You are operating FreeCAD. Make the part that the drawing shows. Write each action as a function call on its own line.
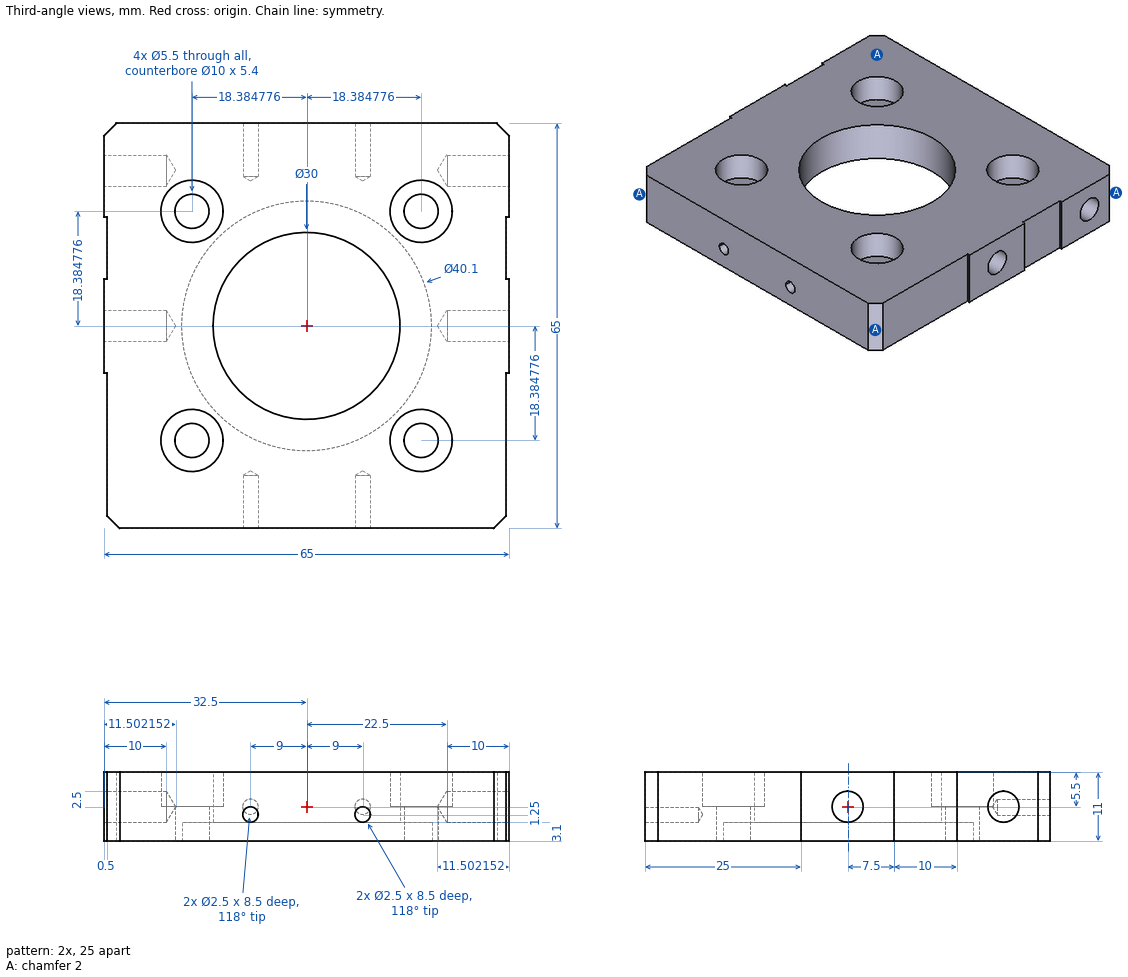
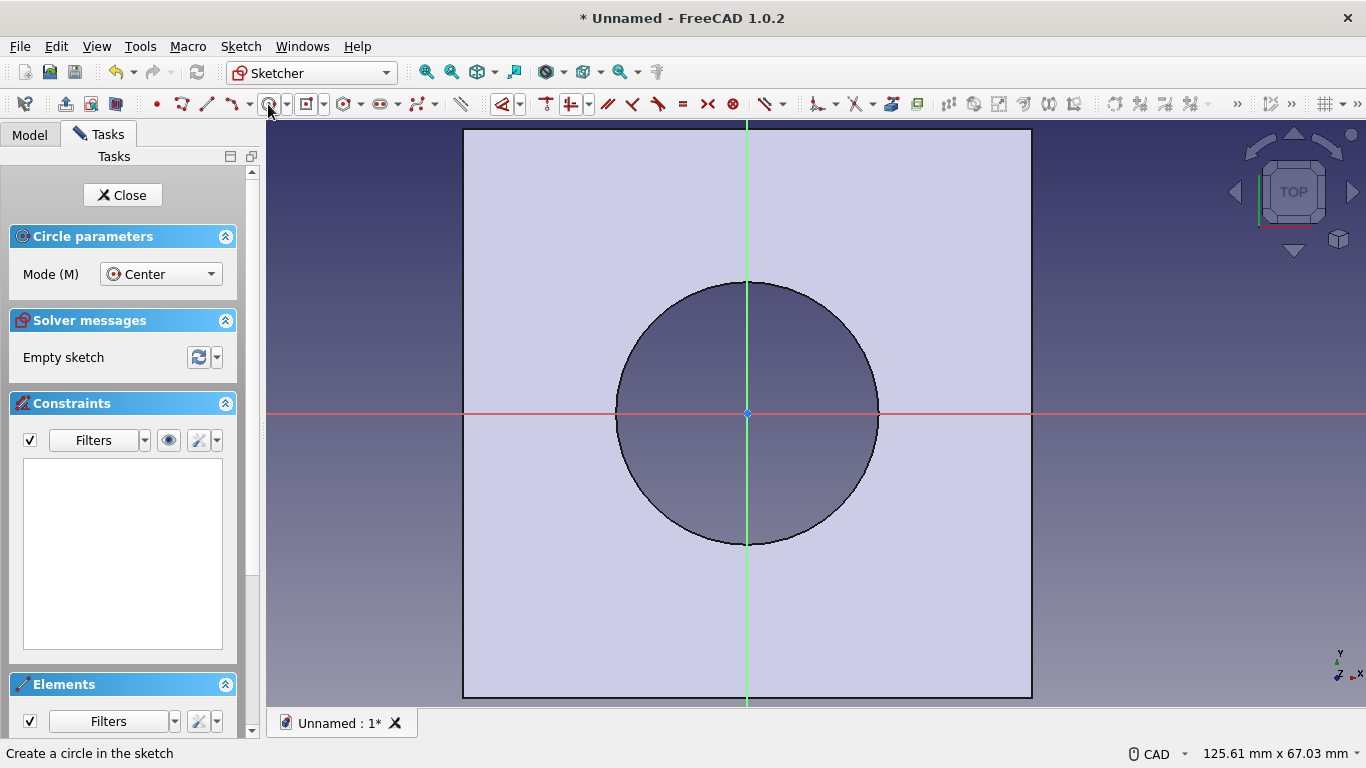
click(586, 253)
click(603, 235)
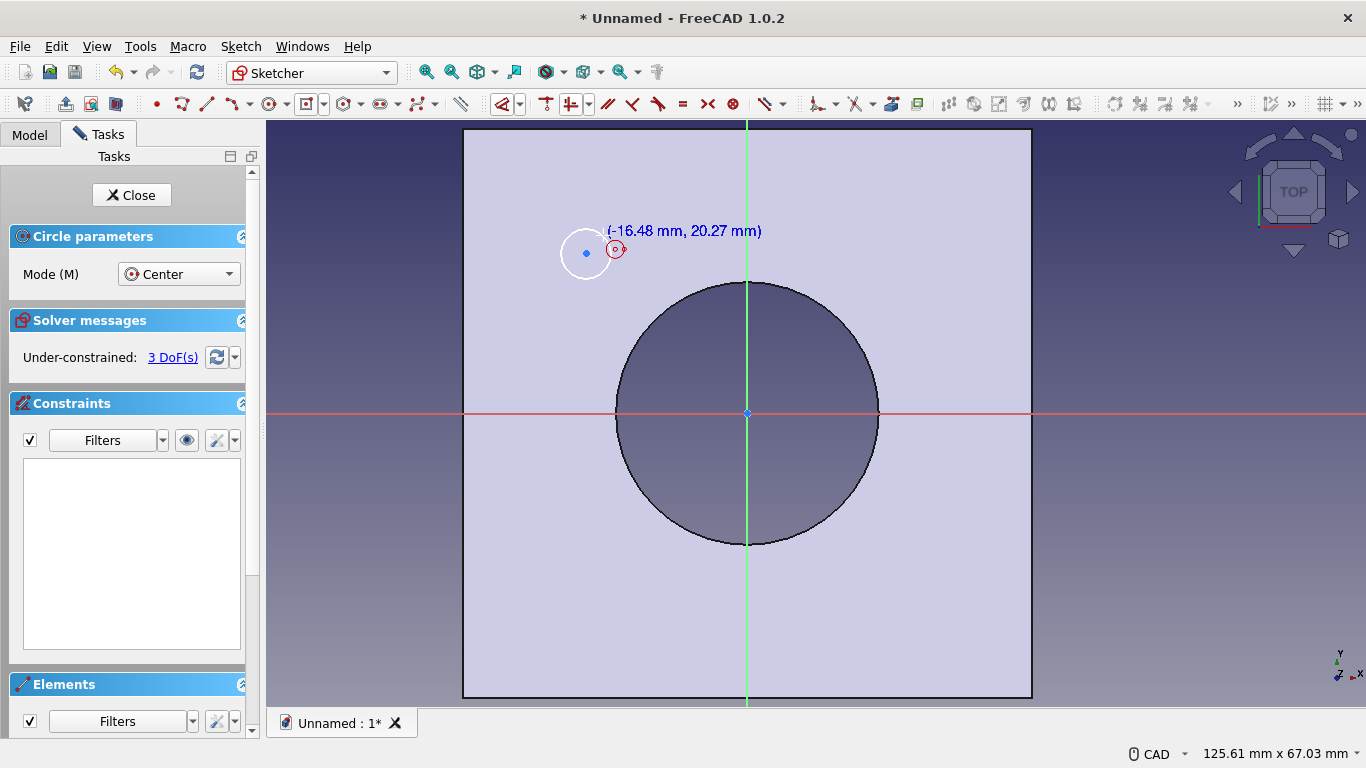
click(908, 253)
click(925, 235)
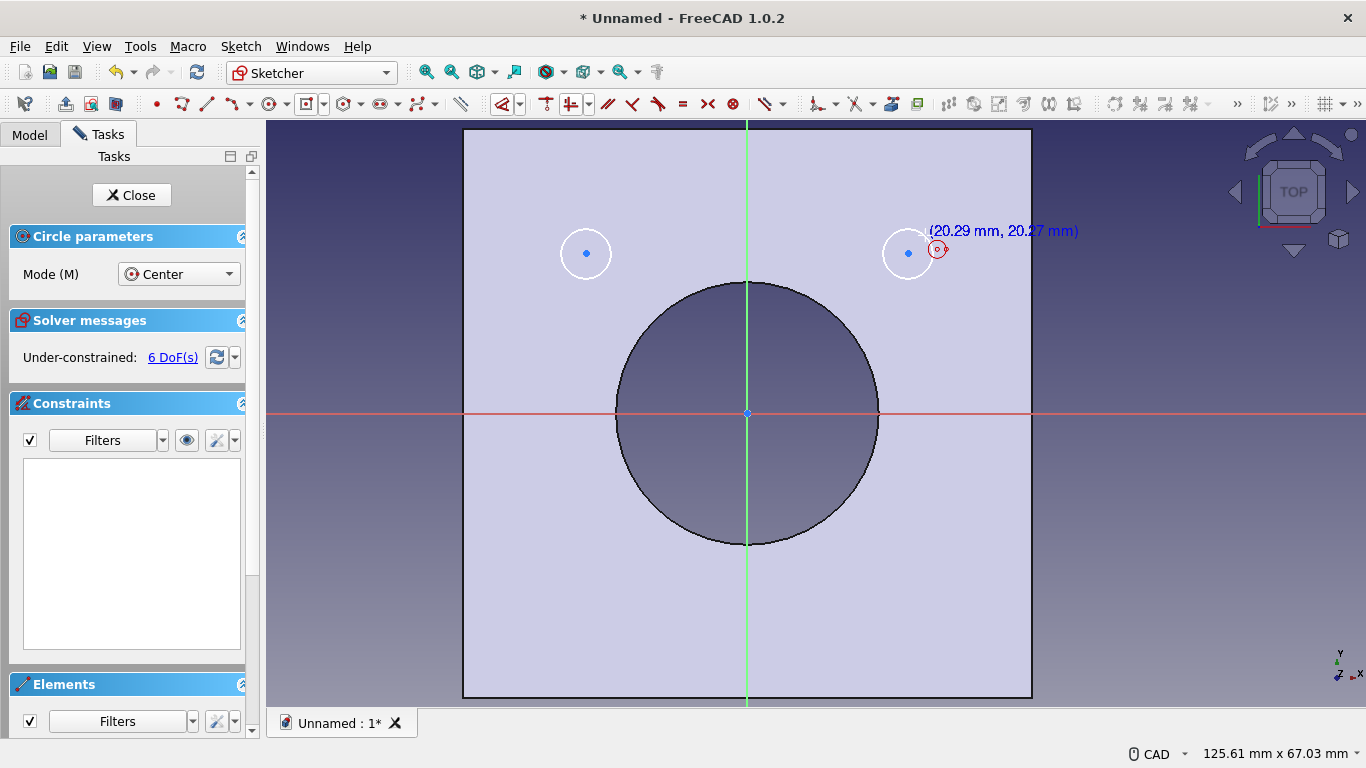
click(908, 574)
click(925, 557)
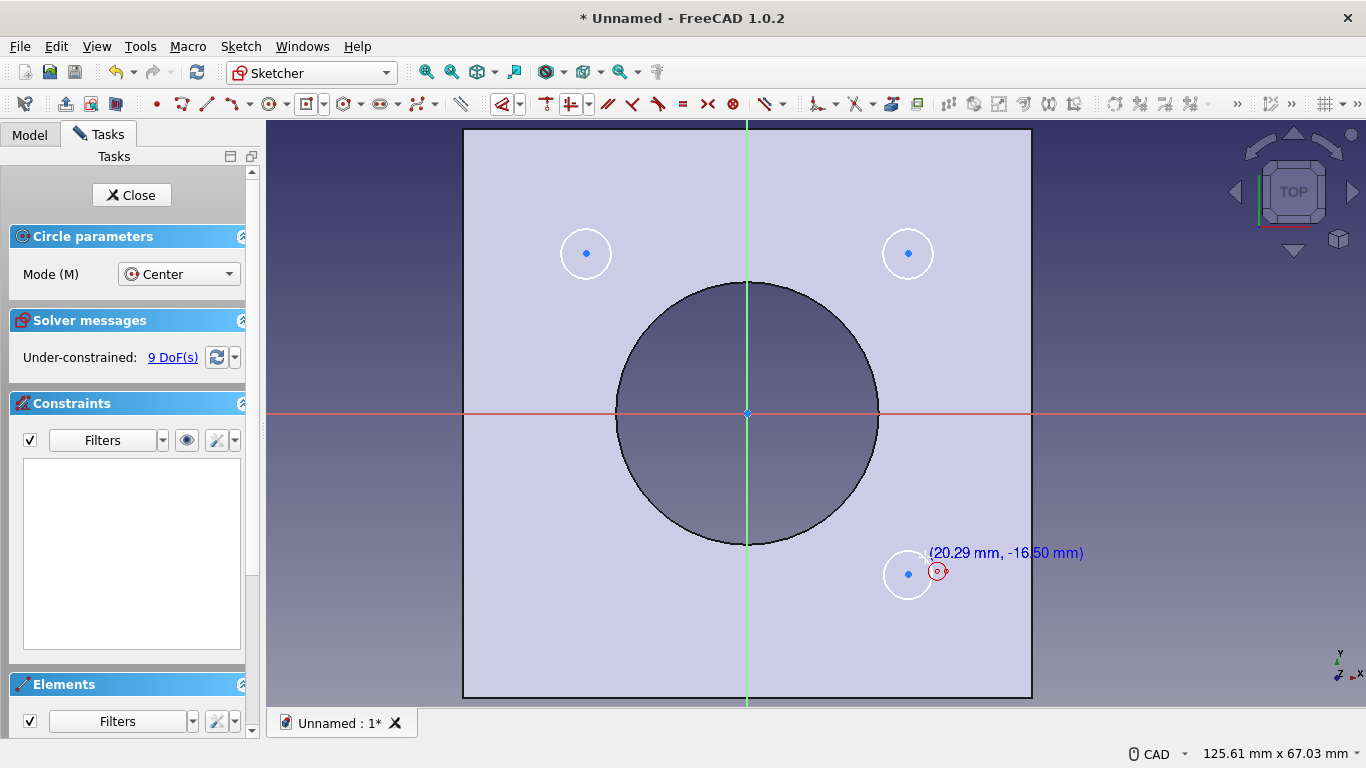
click(586, 574)
click(603, 557)
key(Escape)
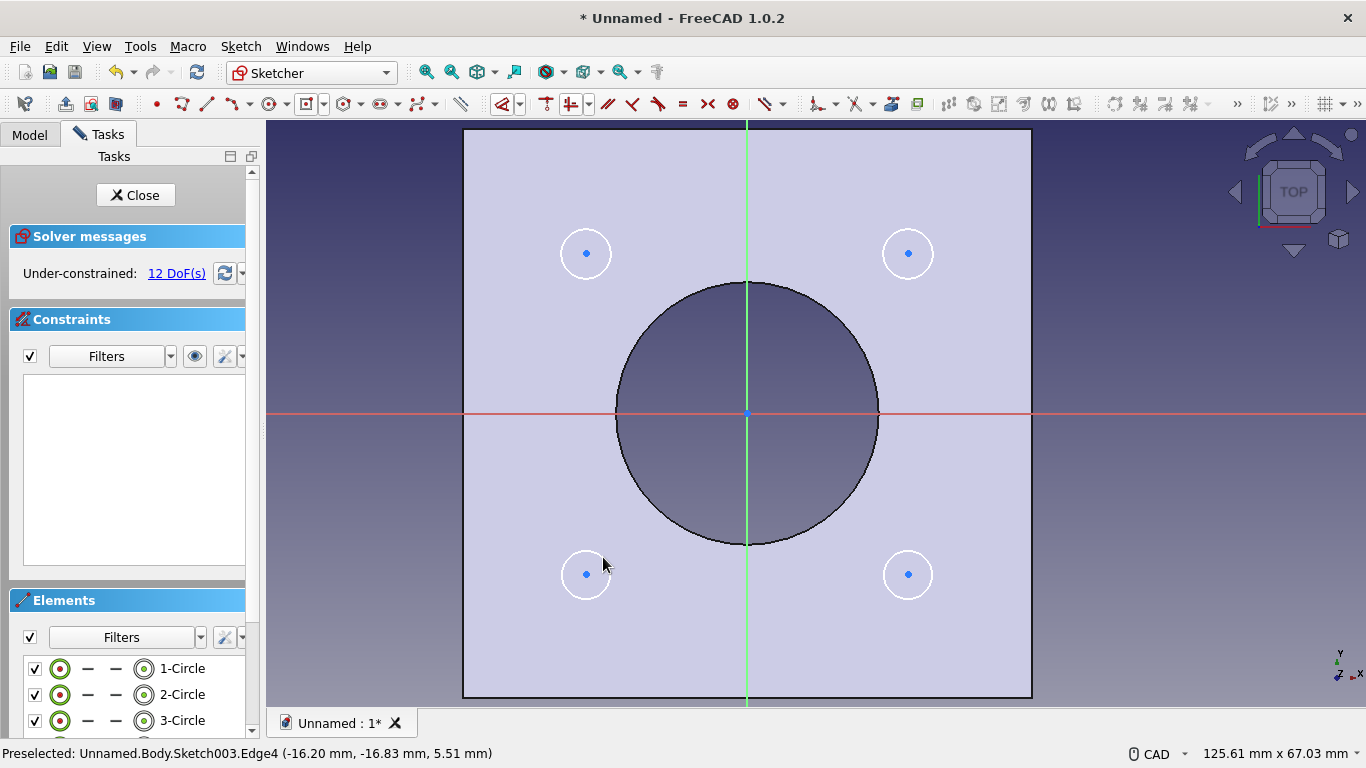
click(603, 236)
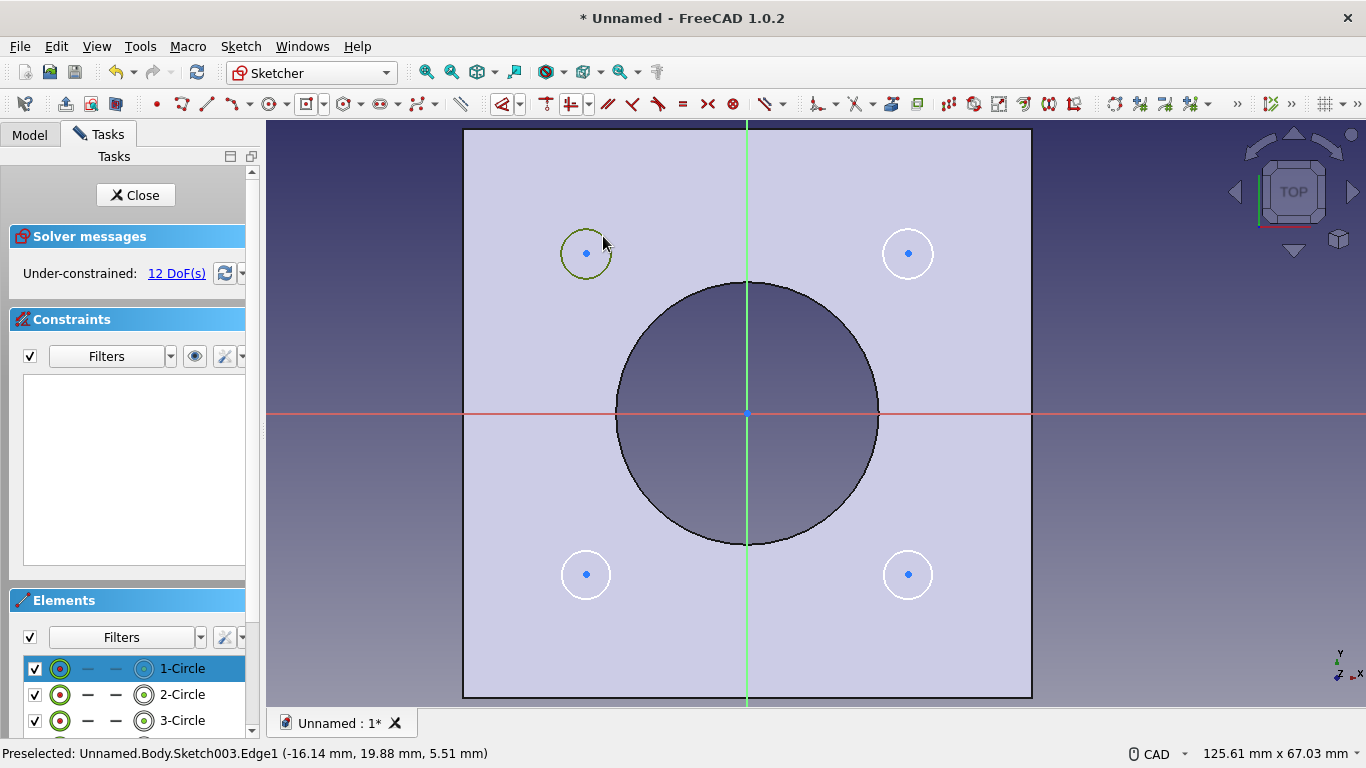
click(925, 236)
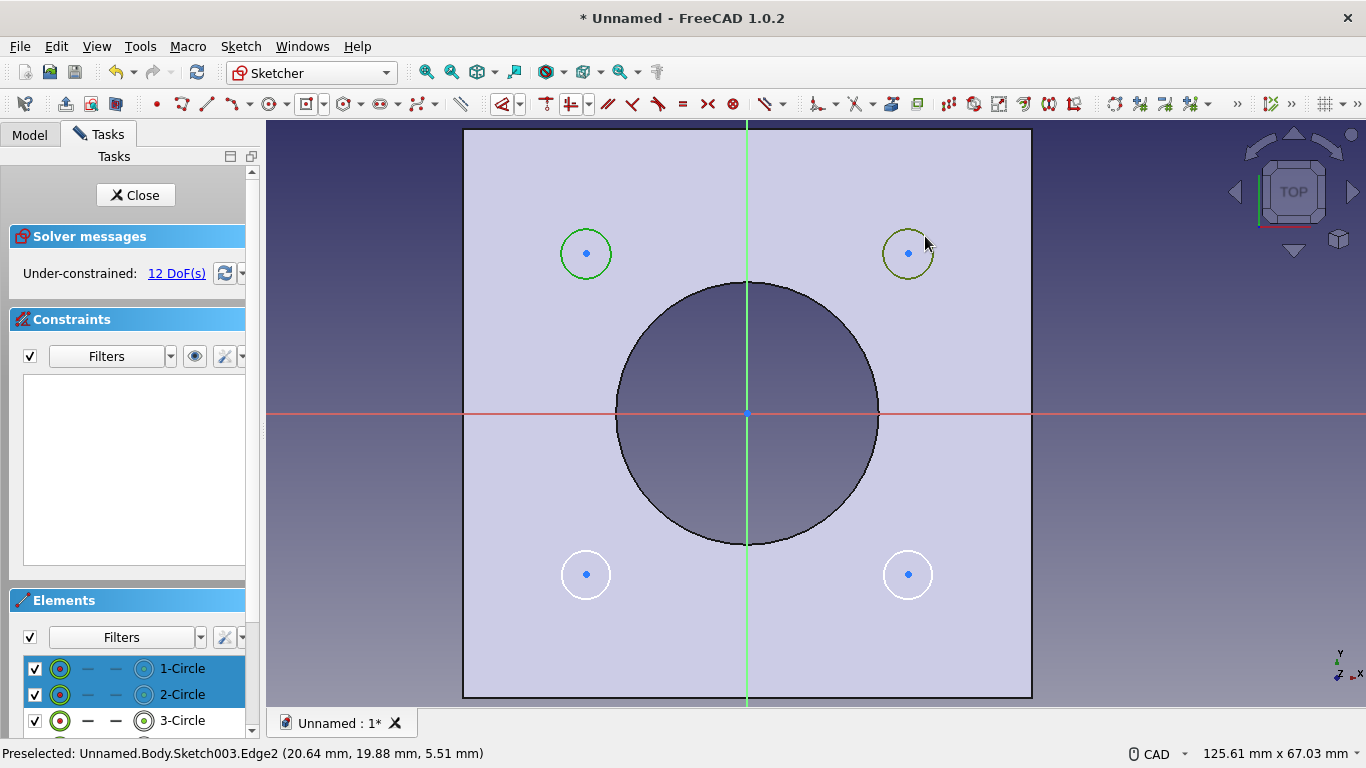
click(925, 558)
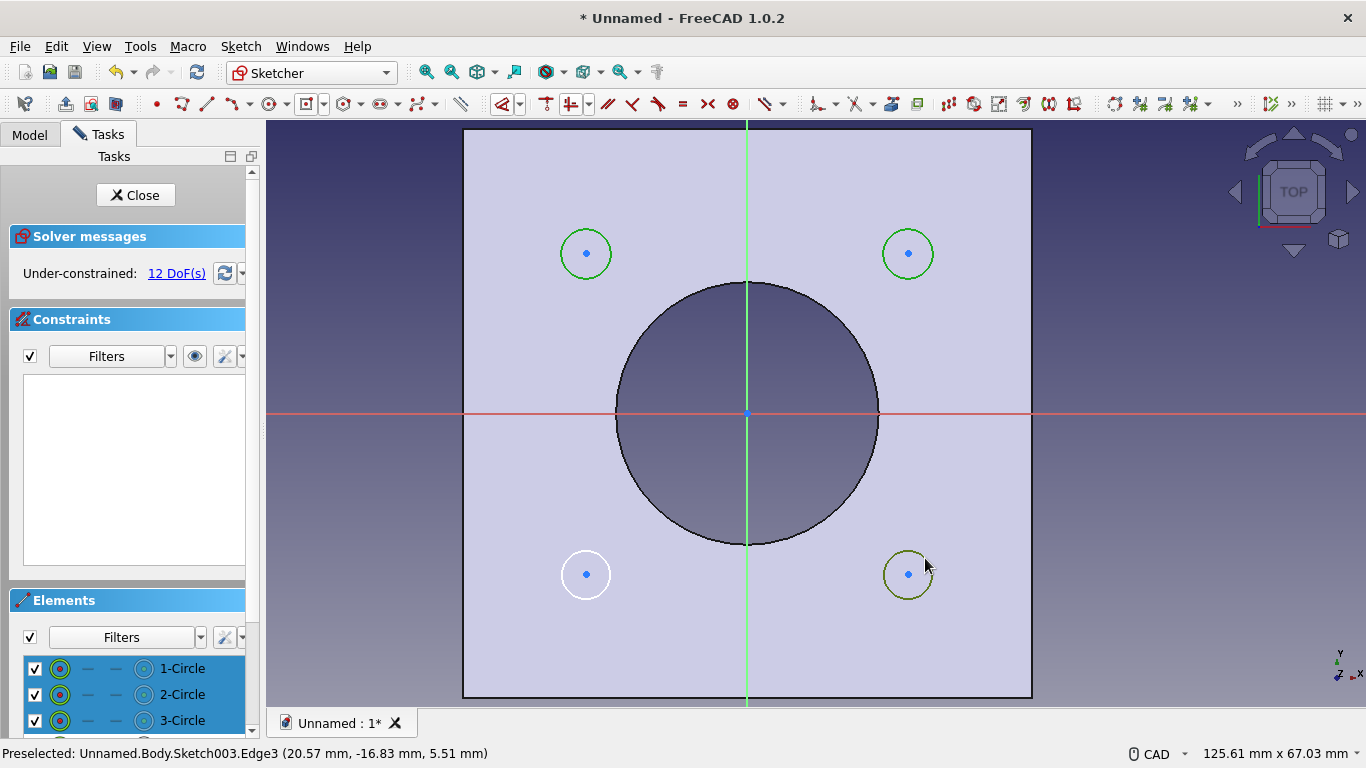
click(603, 558)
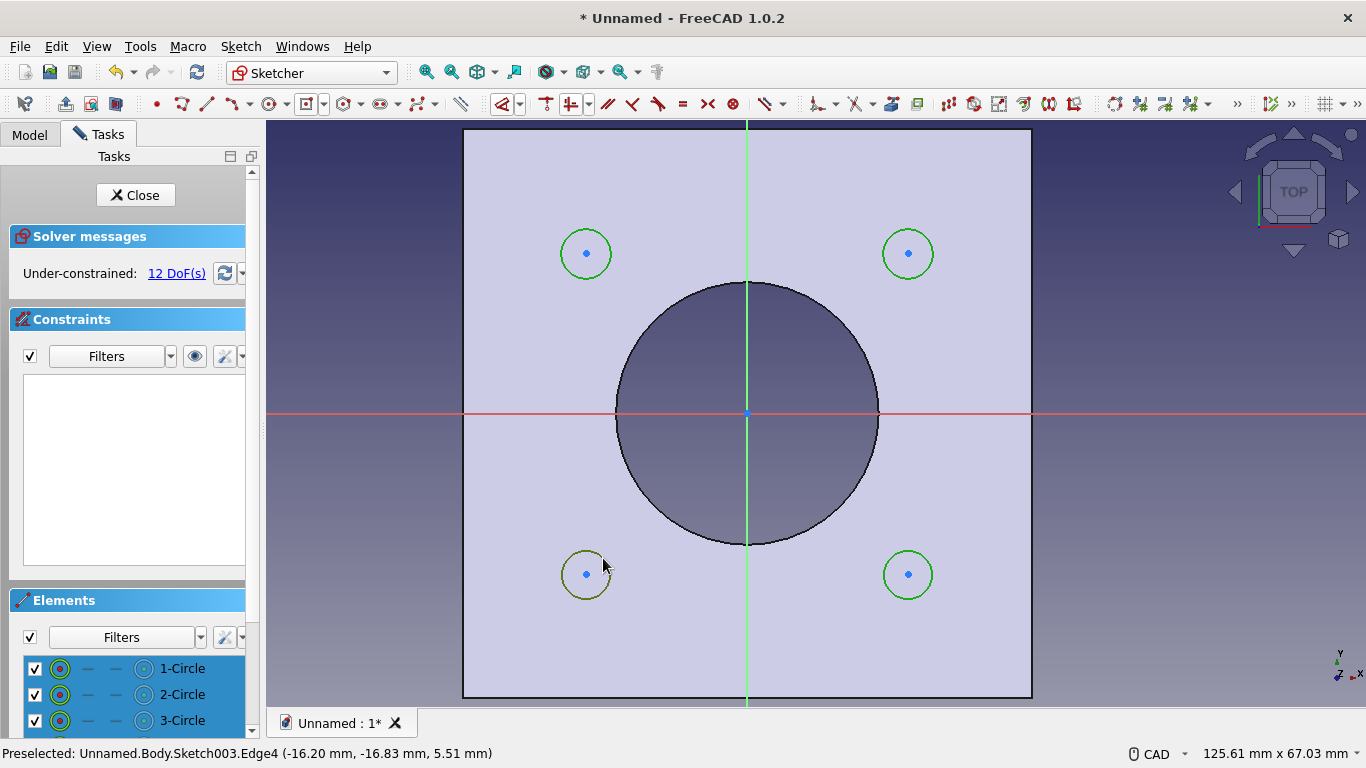
click(683, 104)